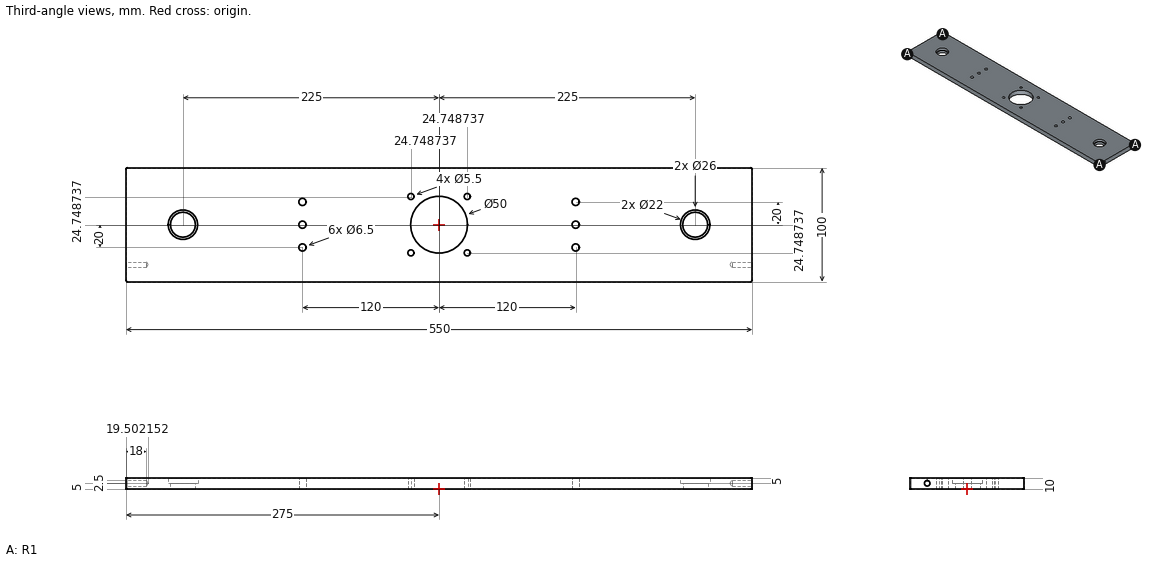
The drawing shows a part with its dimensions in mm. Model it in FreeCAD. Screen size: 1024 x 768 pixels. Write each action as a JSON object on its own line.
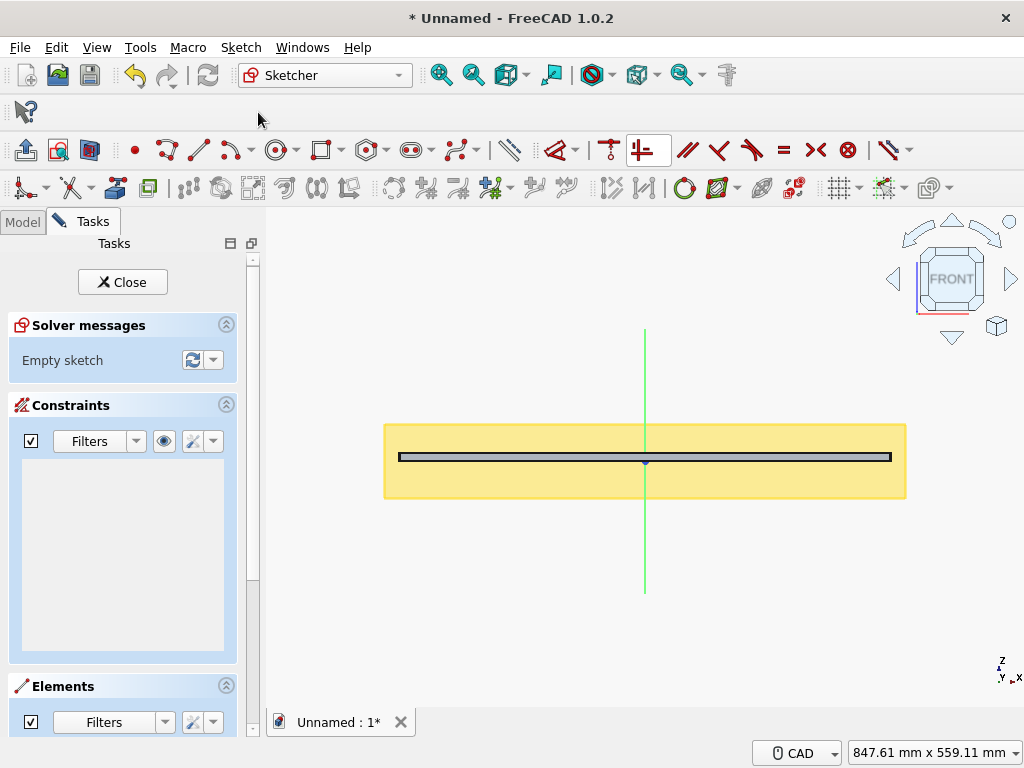
{"action": "key", "text": "q s"}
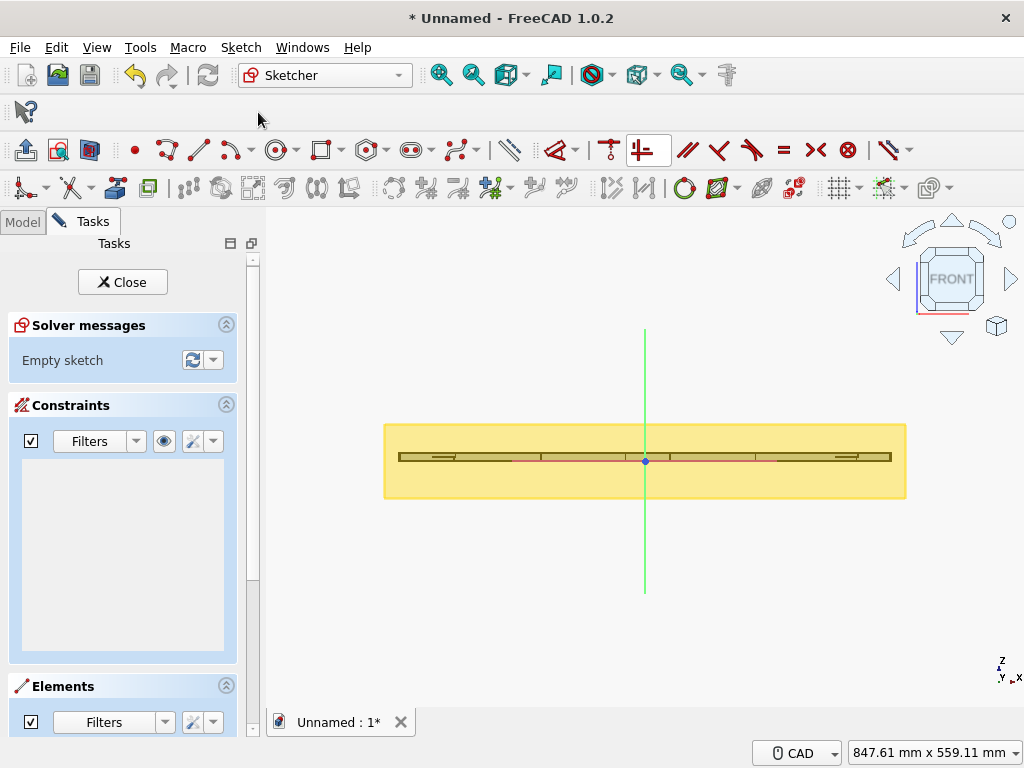
{"action": "scroll", "coordinate": [401, 456], "scroll_direction": "up", "scroll_amount": 14}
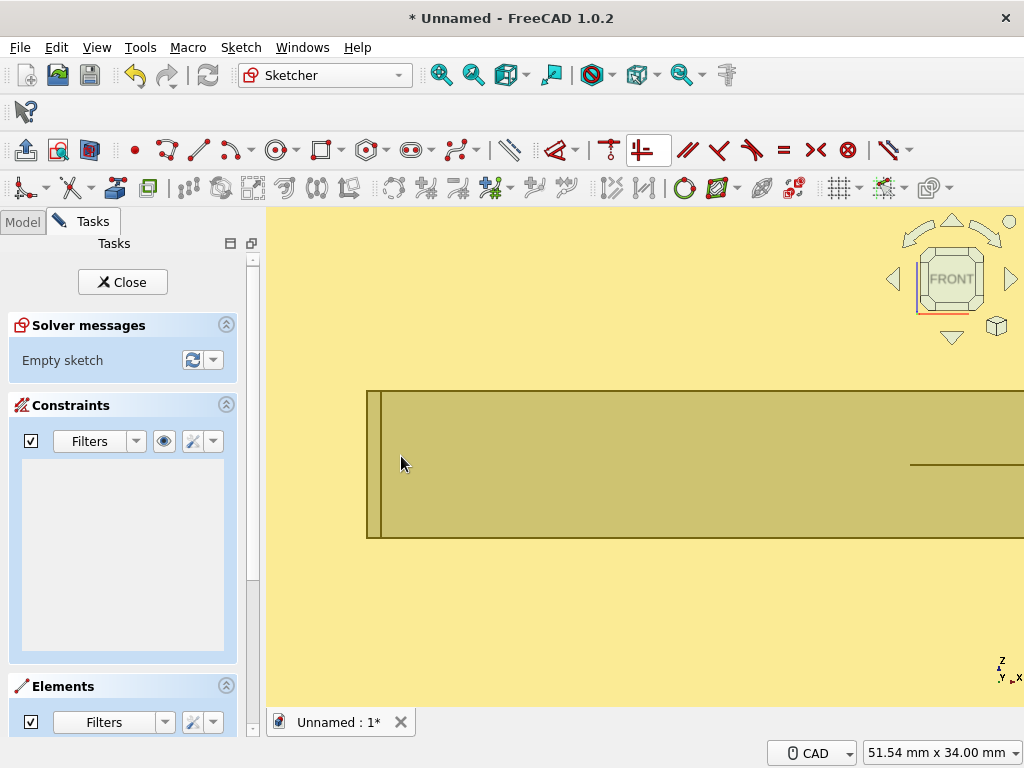
{"action": "left_click", "coordinate": [168, 150]}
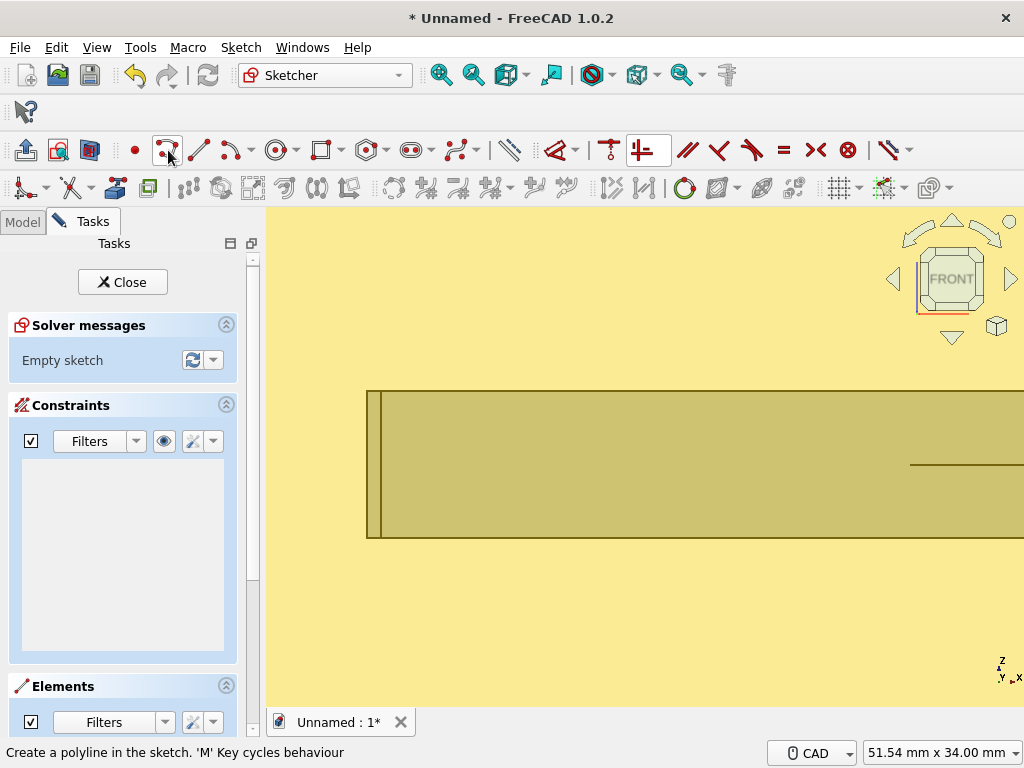
{"action": "left_click", "coordinate": [653, 465]}
{"action": "left_click", "coordinate": [367, 465]}
{"action": "left_click", "coordinate": [367, 428]}
{"action": "left_click", "coordinate": [631, 428]}
{"action": "left_click", "coordinate": [653, 466]}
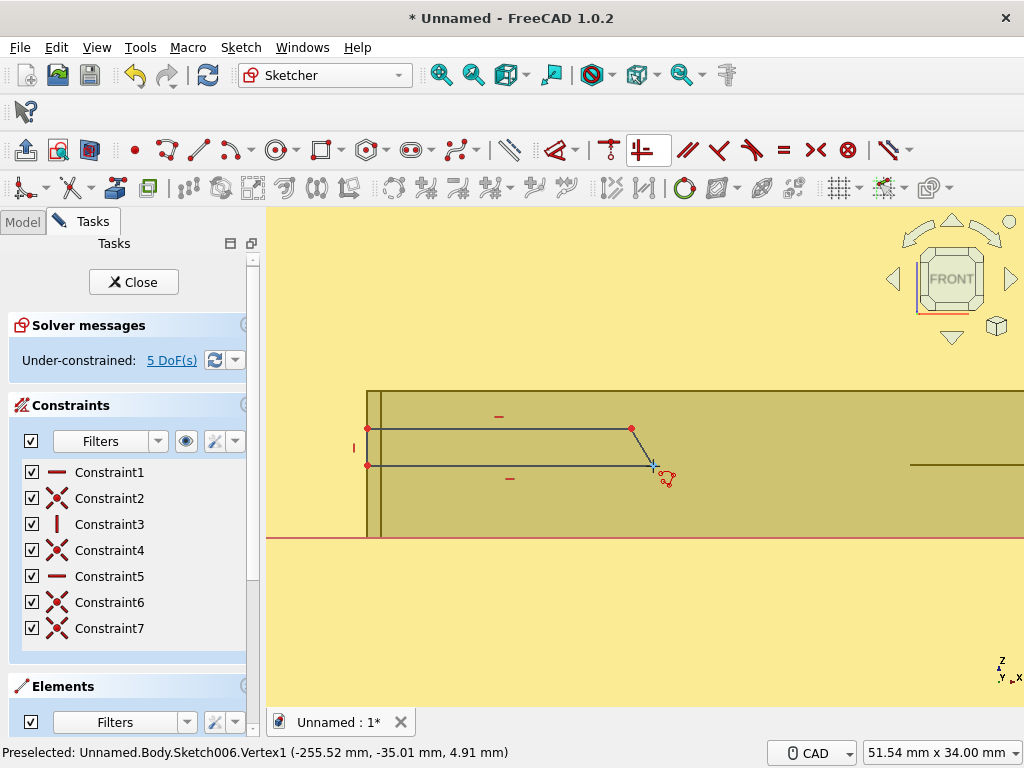
{"action": "key", "text": "g l"}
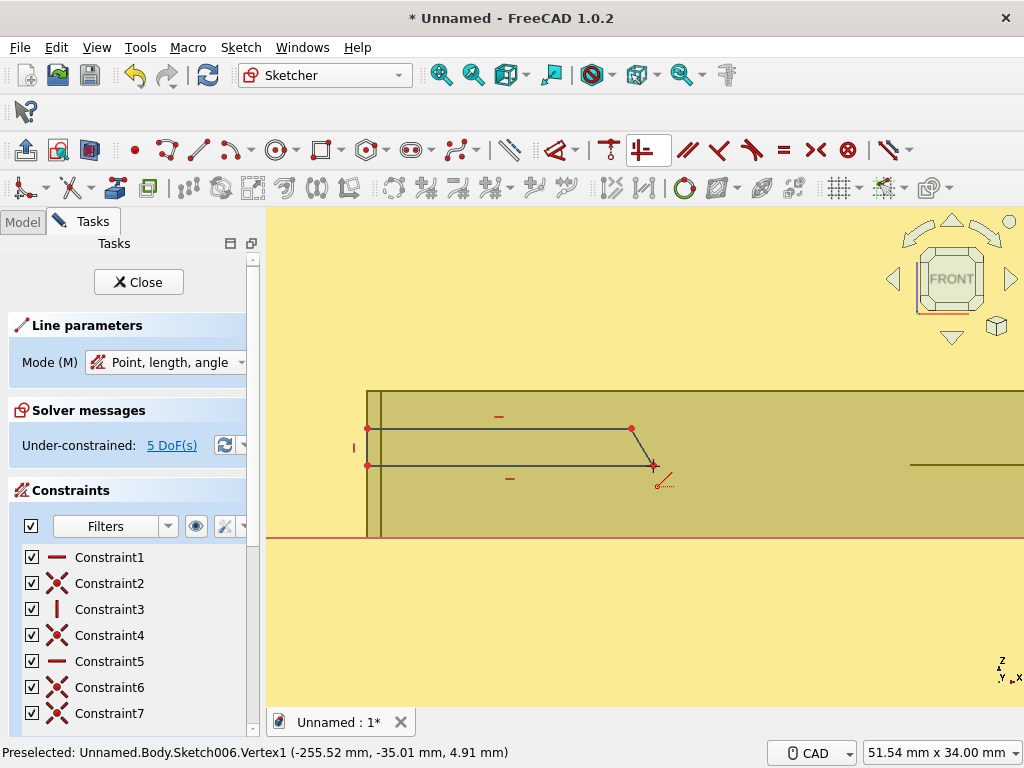
{"action": "left_click", "coordinate": [682, 465]}
{"action": "left_click", "coordinate": [768, 465]}
{"action": "key", "text": "Escape"}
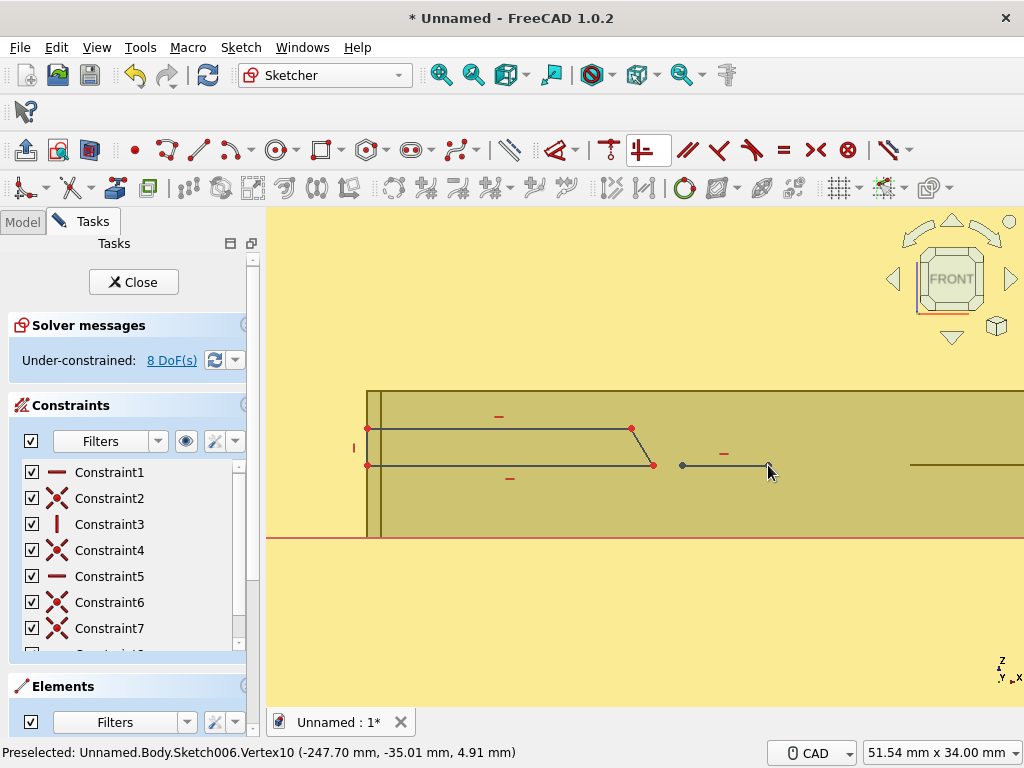
{"action": "left_click", "coordinate": [708, 466]}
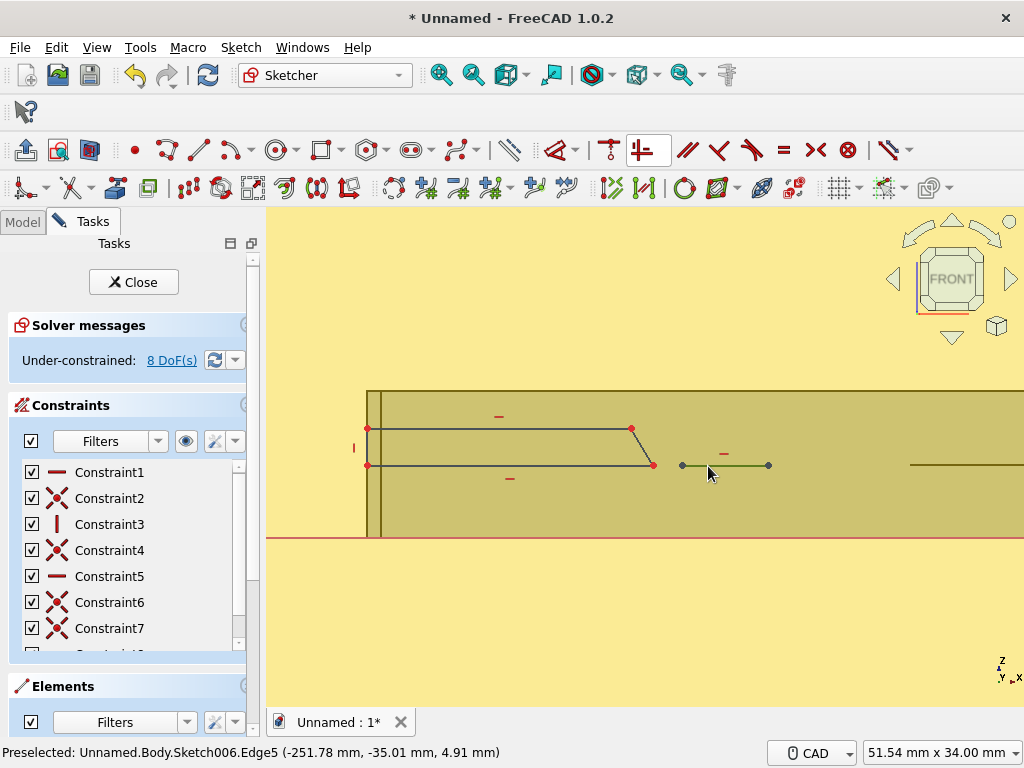
{"action": "key", "text": "g n"}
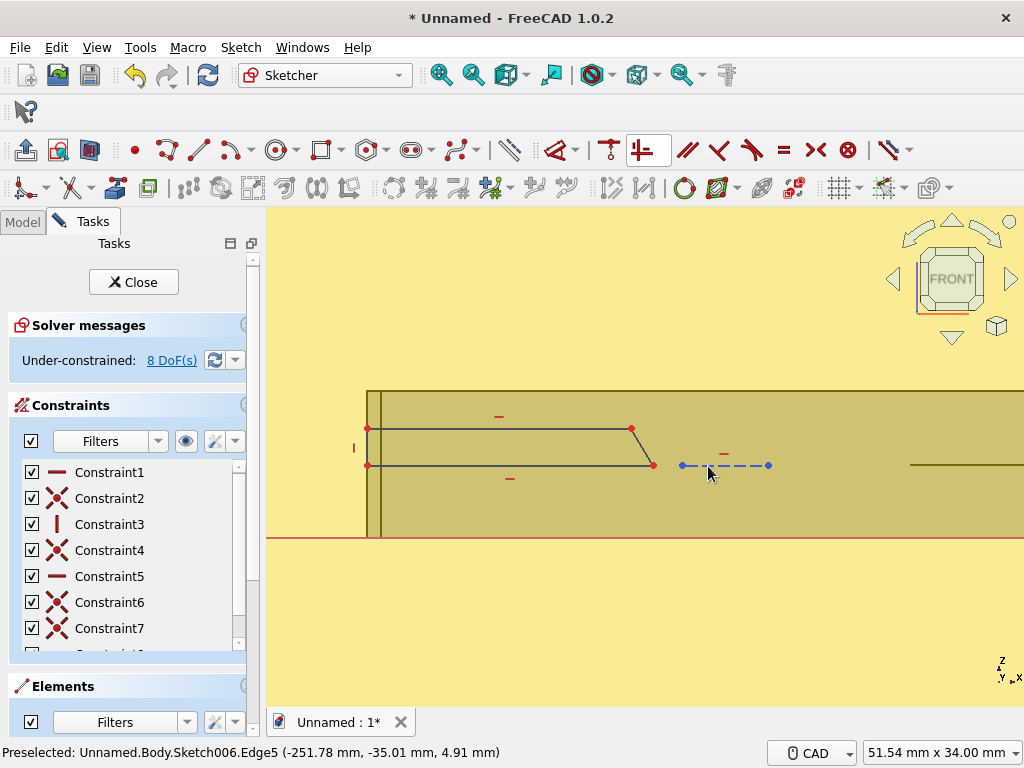
{"action": "key", "text": "d"}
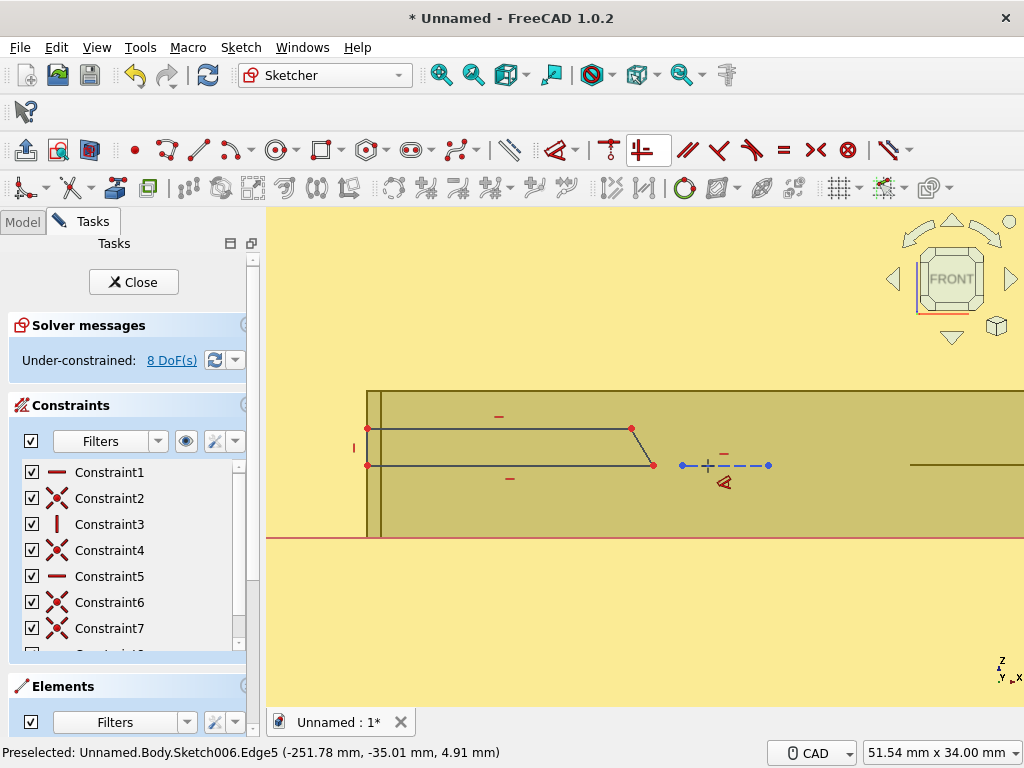
{"action": "left_click", "coordinate": [446, 429]}
{"action": "left_click", "coordinate": [499, 395]}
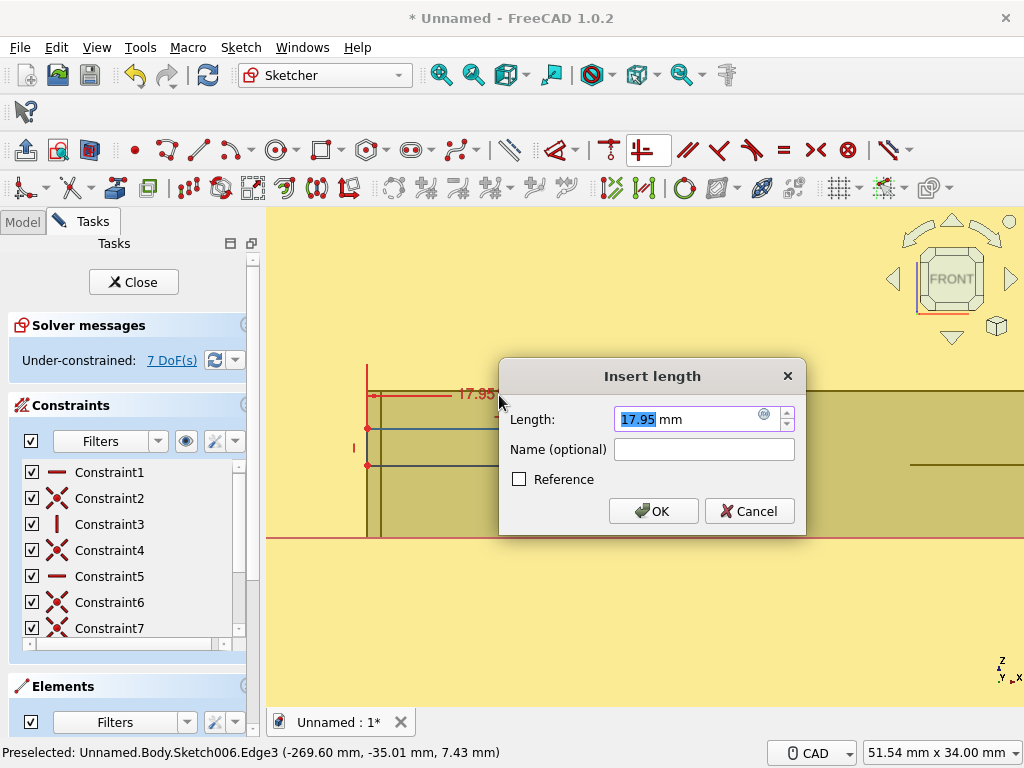
{"action": "type", "text": "18"}
{"action": "key", "text": "Return"}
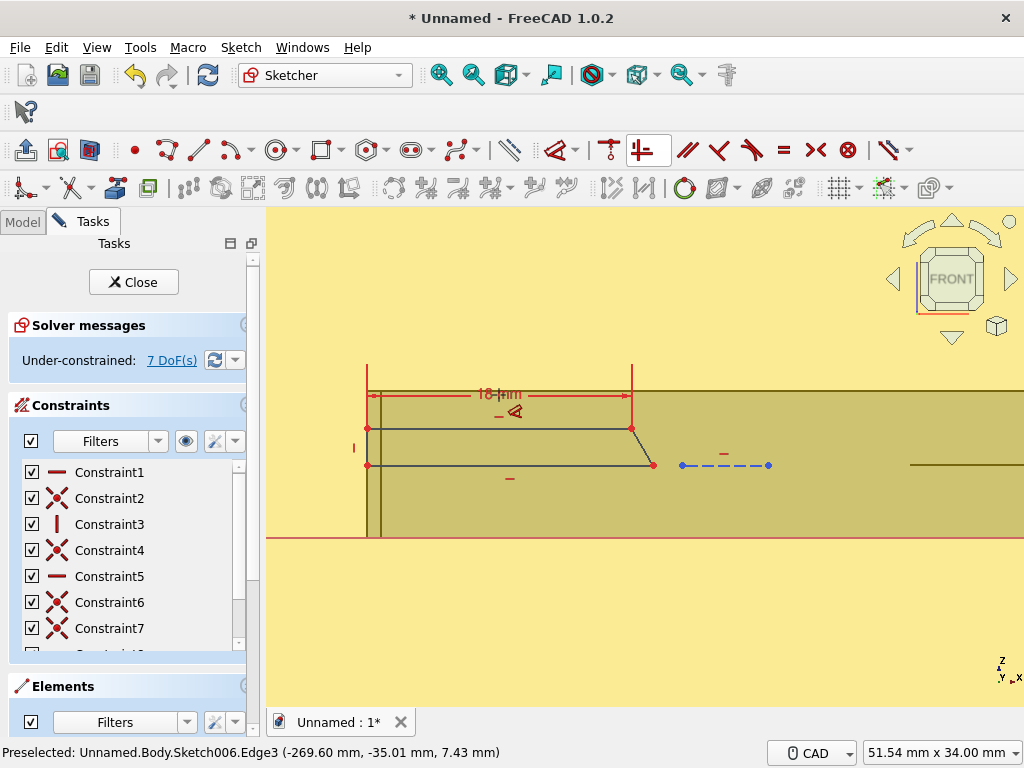
{"action": "left_click", "coordinate": [653, 466]}
{"action": "left_click", "coordinate": [619, 502]}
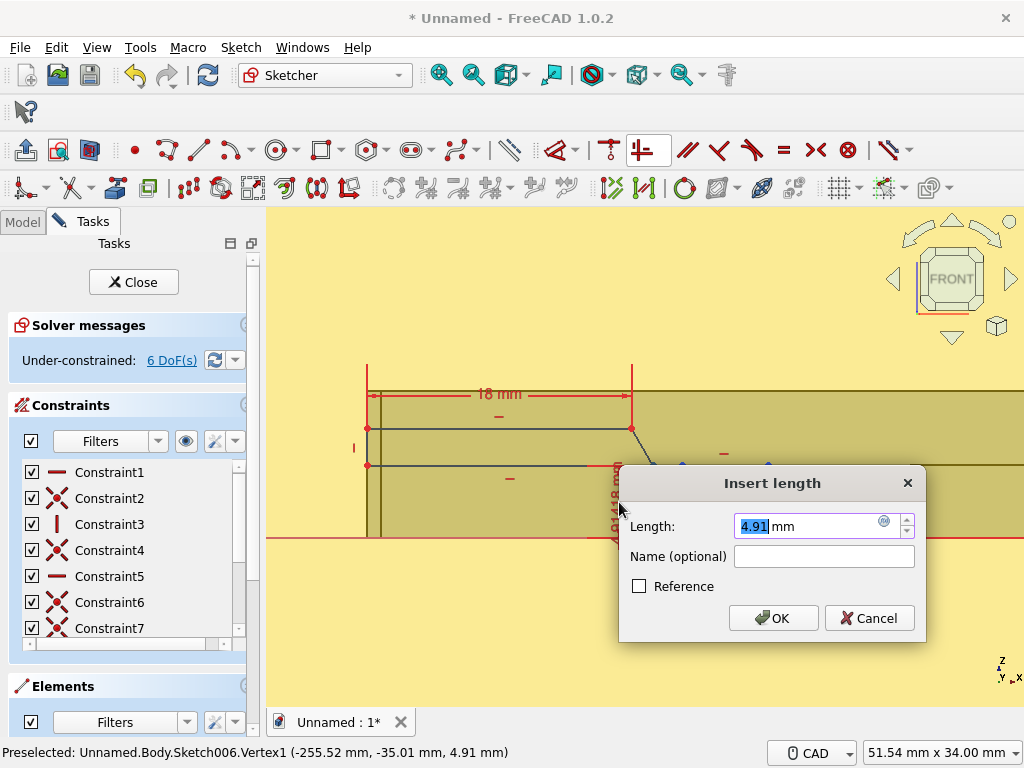
{"action": "type", "text": "5"}
{"action": "key", "text": "Return"}